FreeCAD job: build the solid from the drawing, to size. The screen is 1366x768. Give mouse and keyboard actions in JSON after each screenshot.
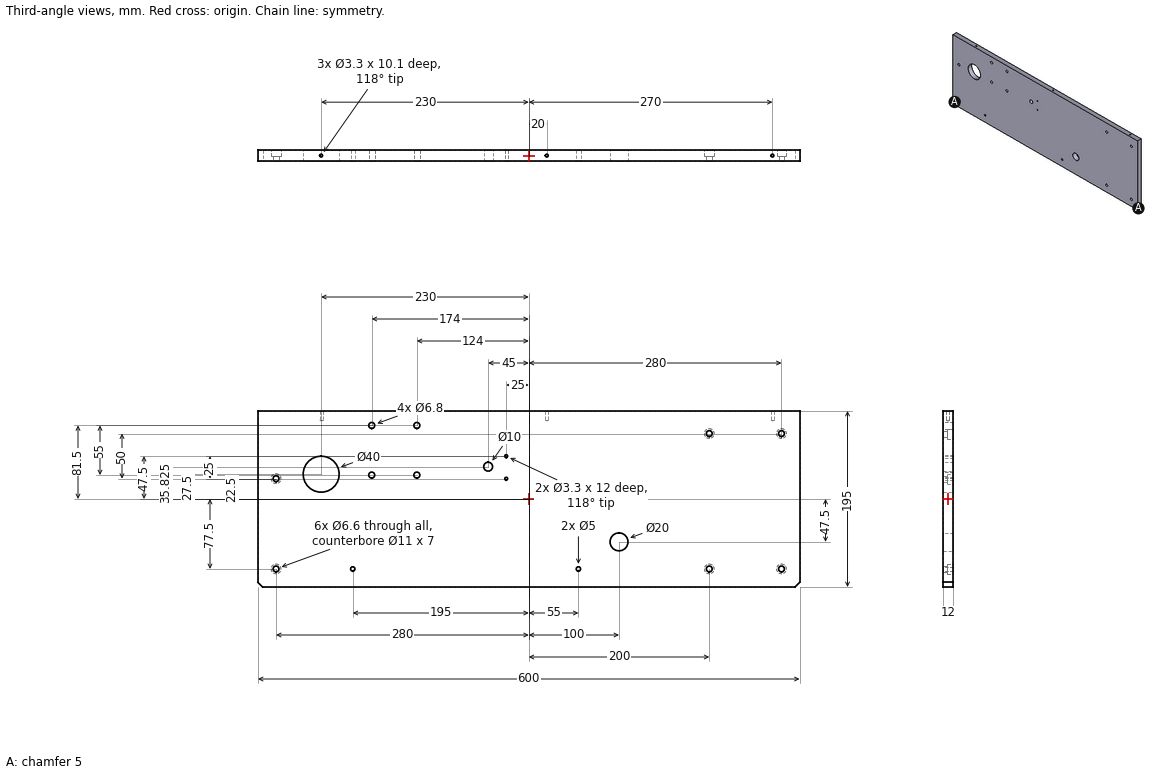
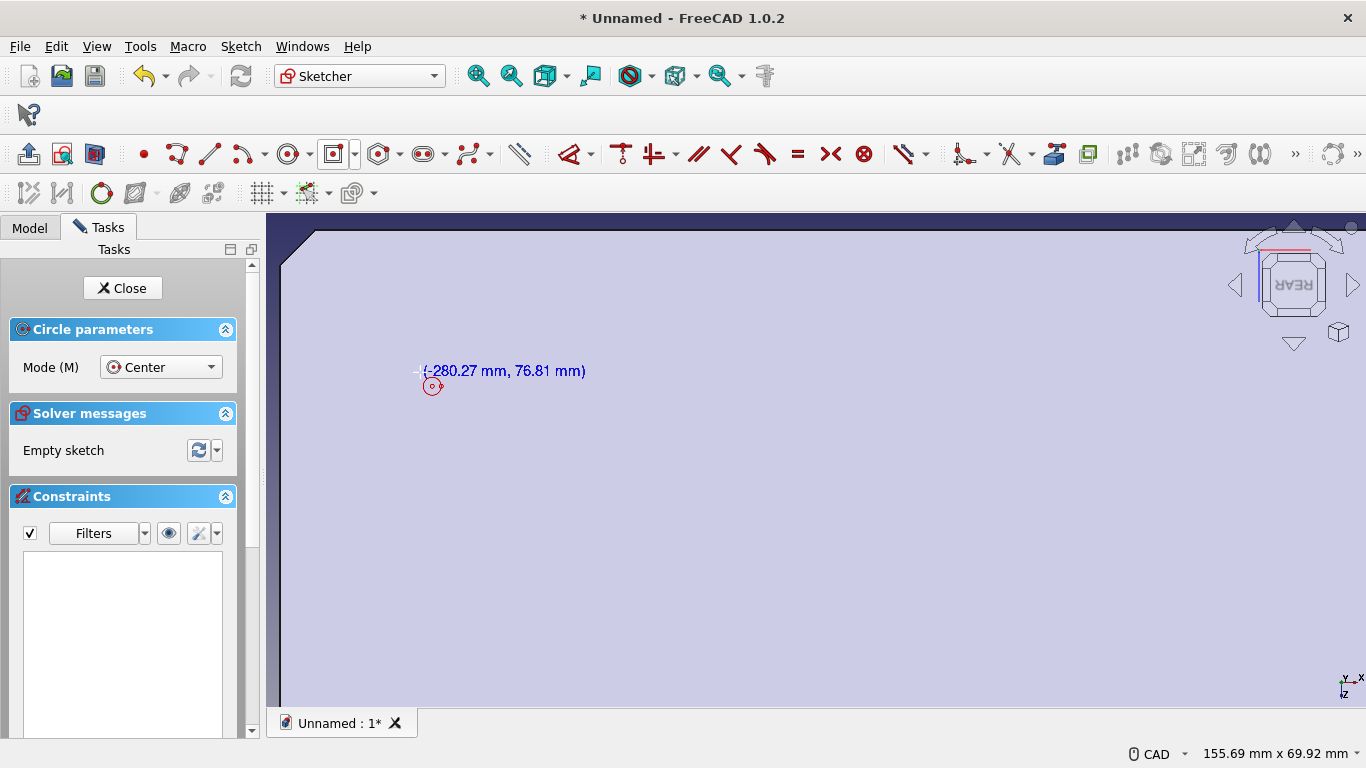
{"action": "scroll", "coordinate": [420, 373], "scroll_direction": "down", "scroll_amount": 9}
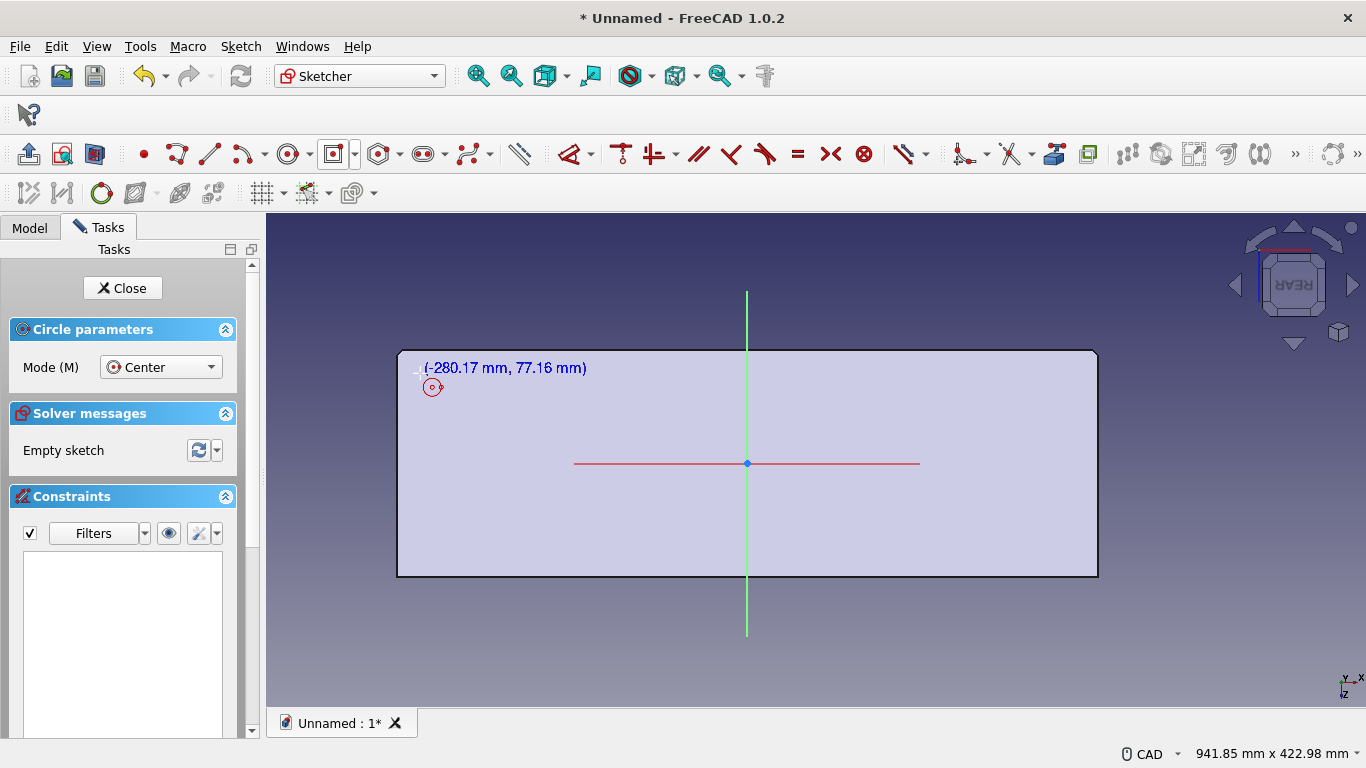
{"action": "left_click", "coordinate": [420, 373]}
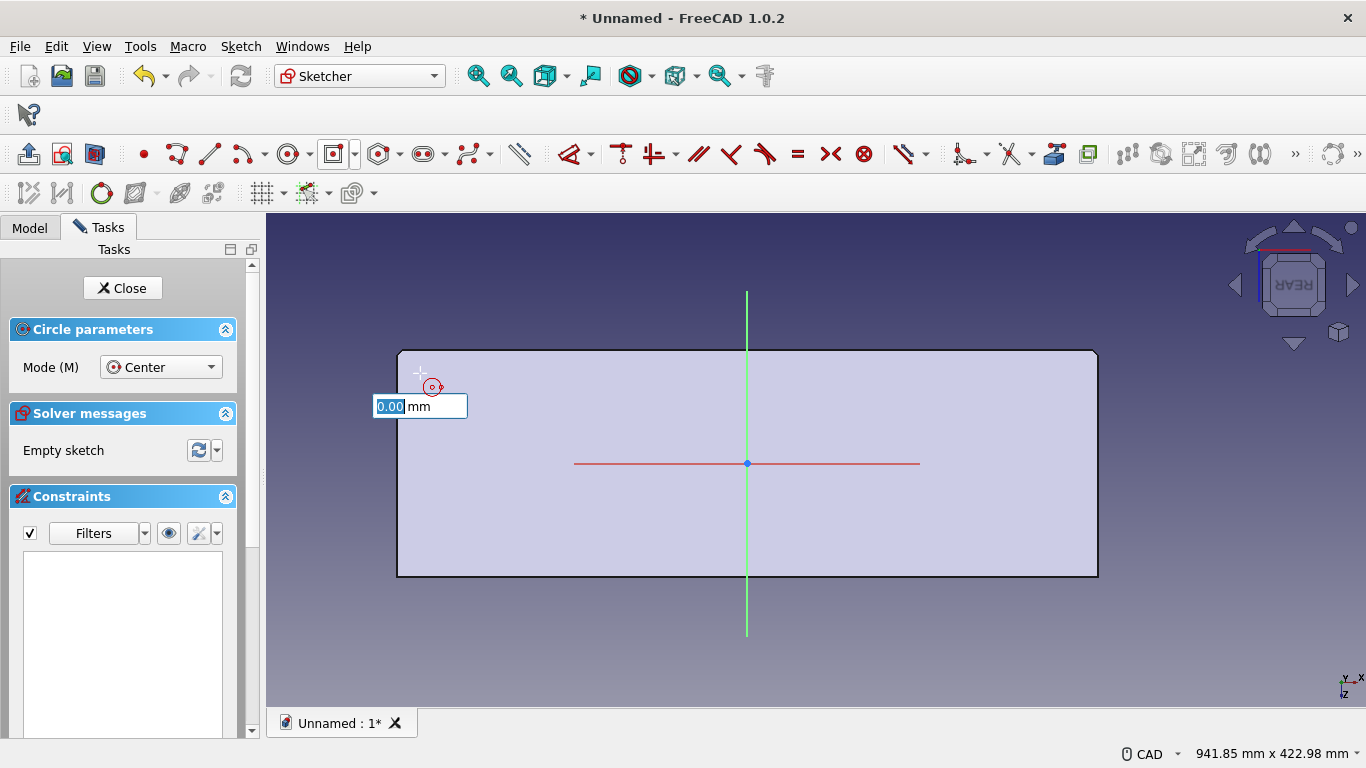
{"action": "scroll", "coordinate": [423, 370], "scroll_direction": "up", "scroll_amount": 8}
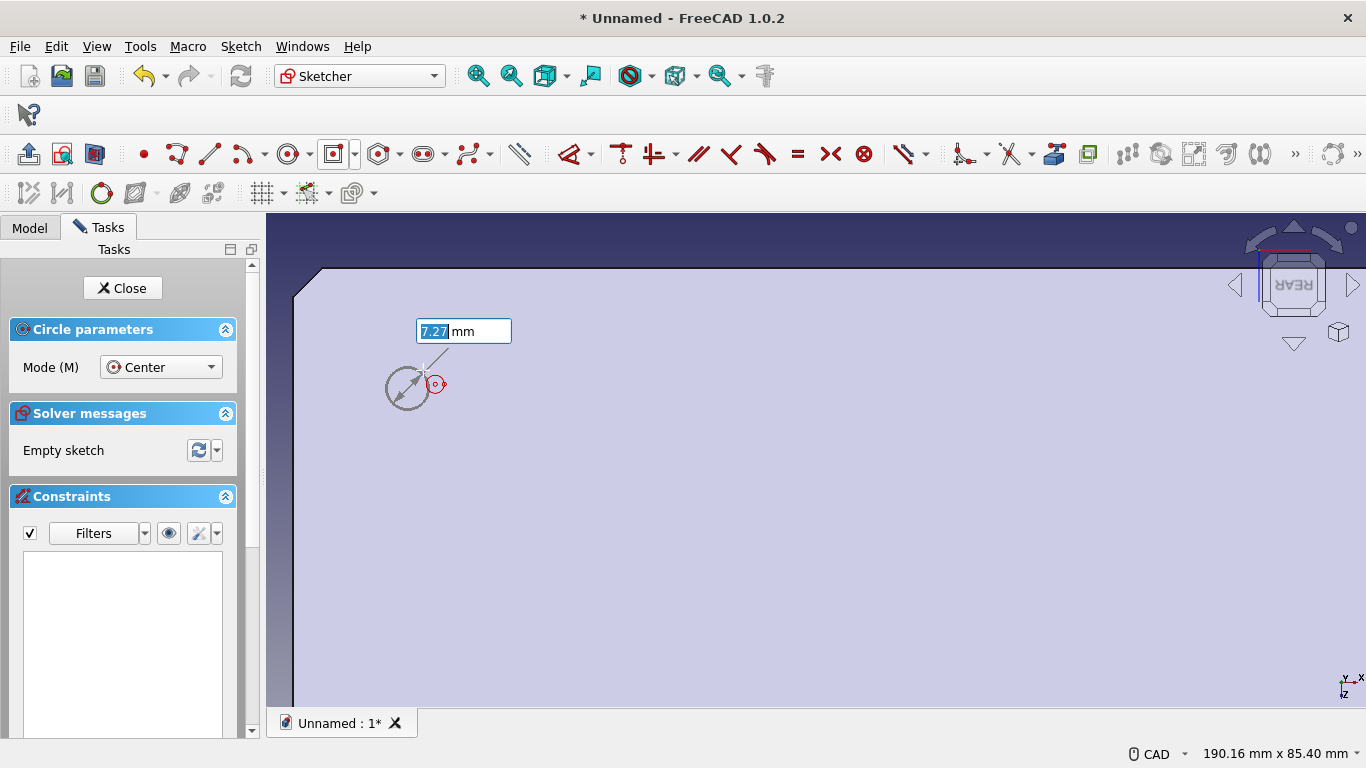
{"action": "left_click", "coordinate": [423, 370]}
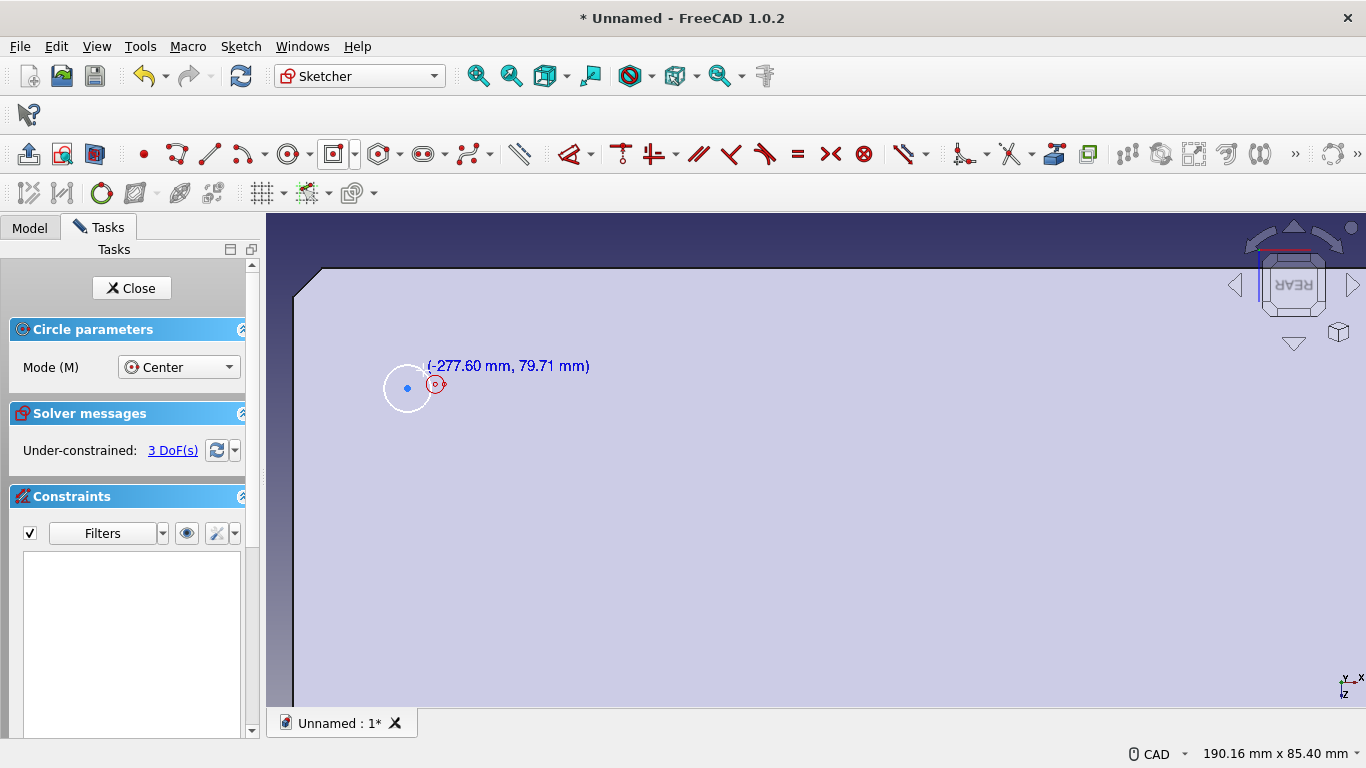
{"action": "scroll", "coordinate": [423, 370], "scroll_direction": "down", "scroll_amount": 8}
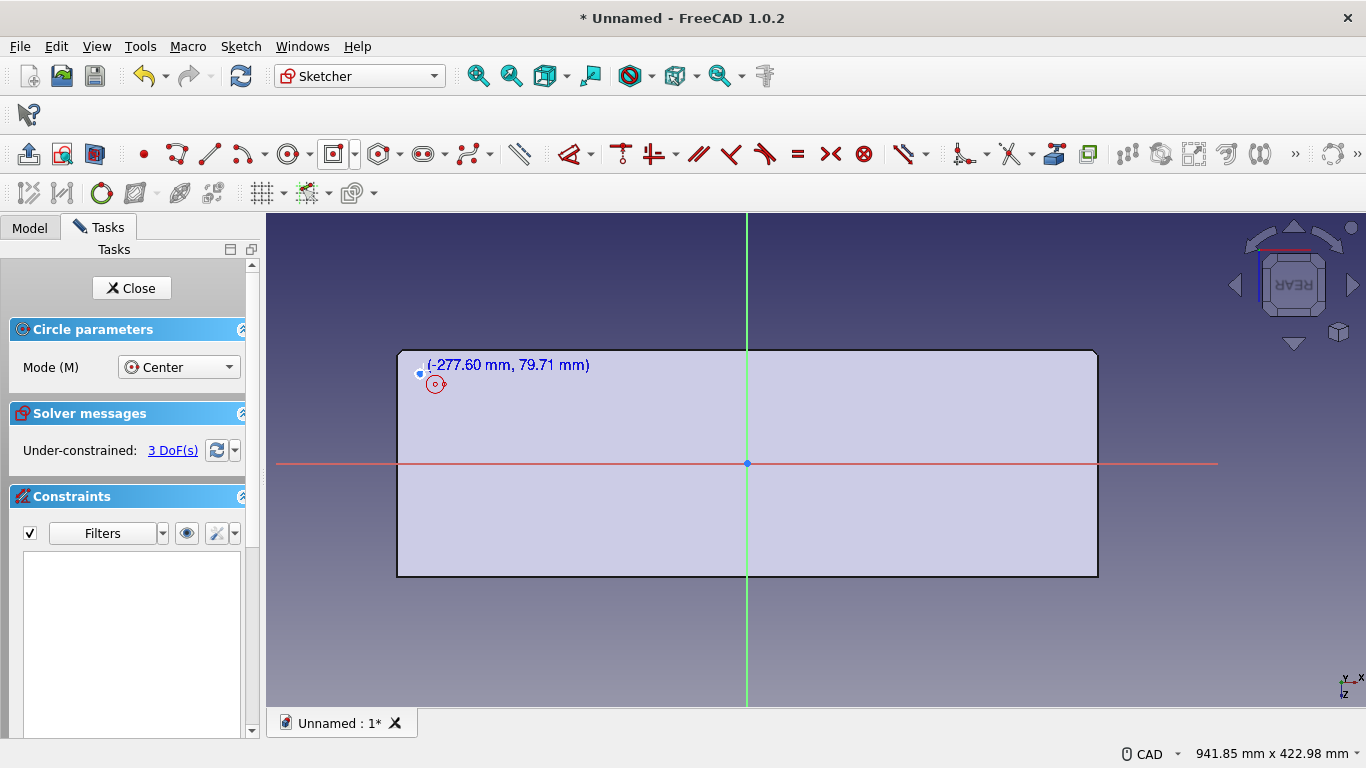
{"action": "scroll", "coordinate": [420, 490], "scroll_direction": "up", "scroll_amount": 9}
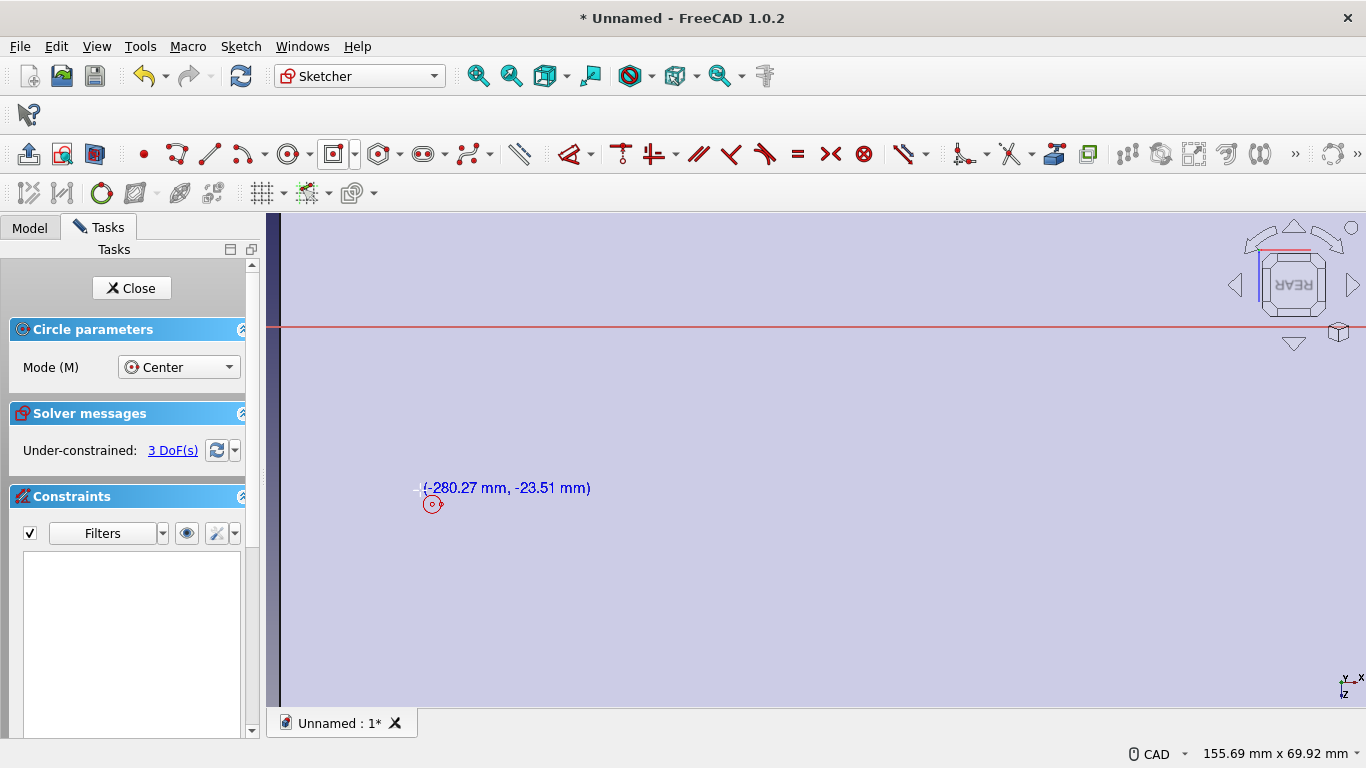
{"action": "scroll", "coordinate": [420, 490], "scroll_direction": "down", "scroll_amount": 9}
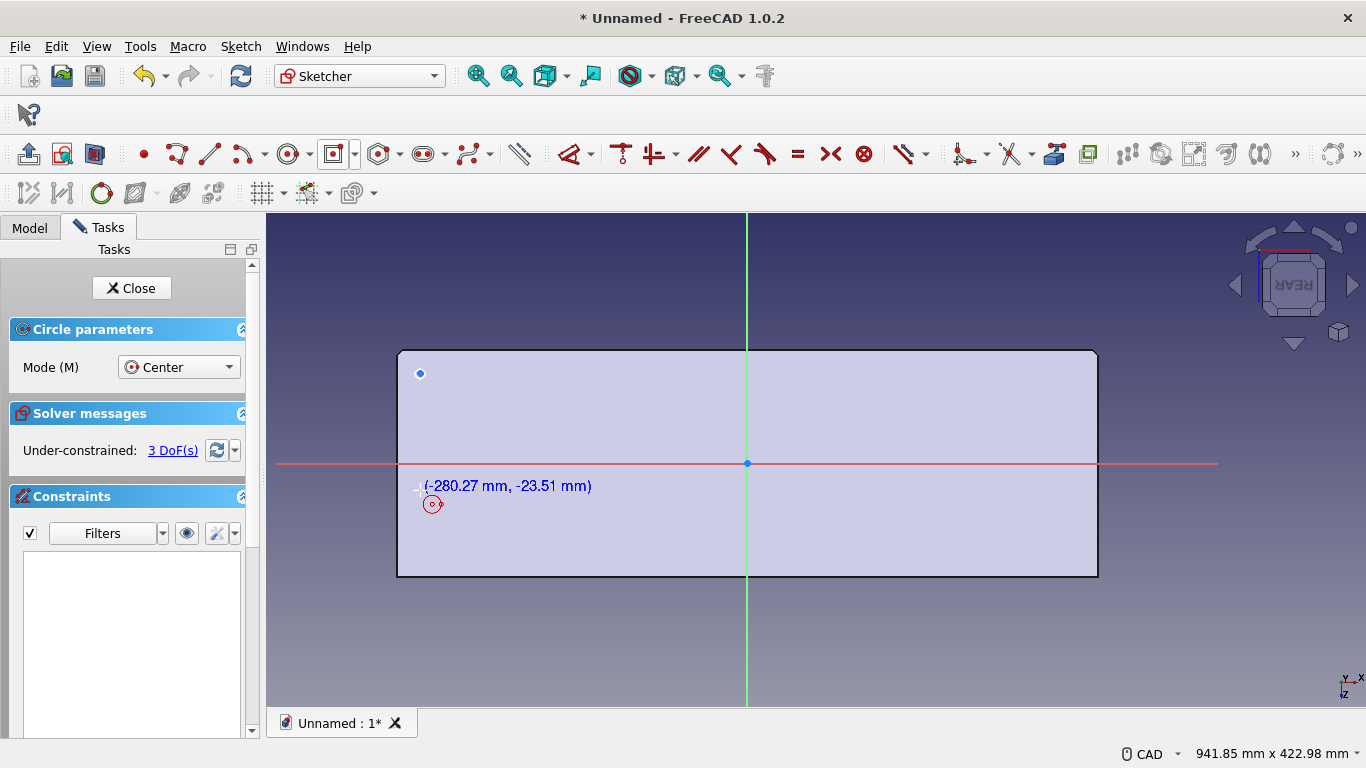
{"action": "left_click", "coordinate": [420, 490]}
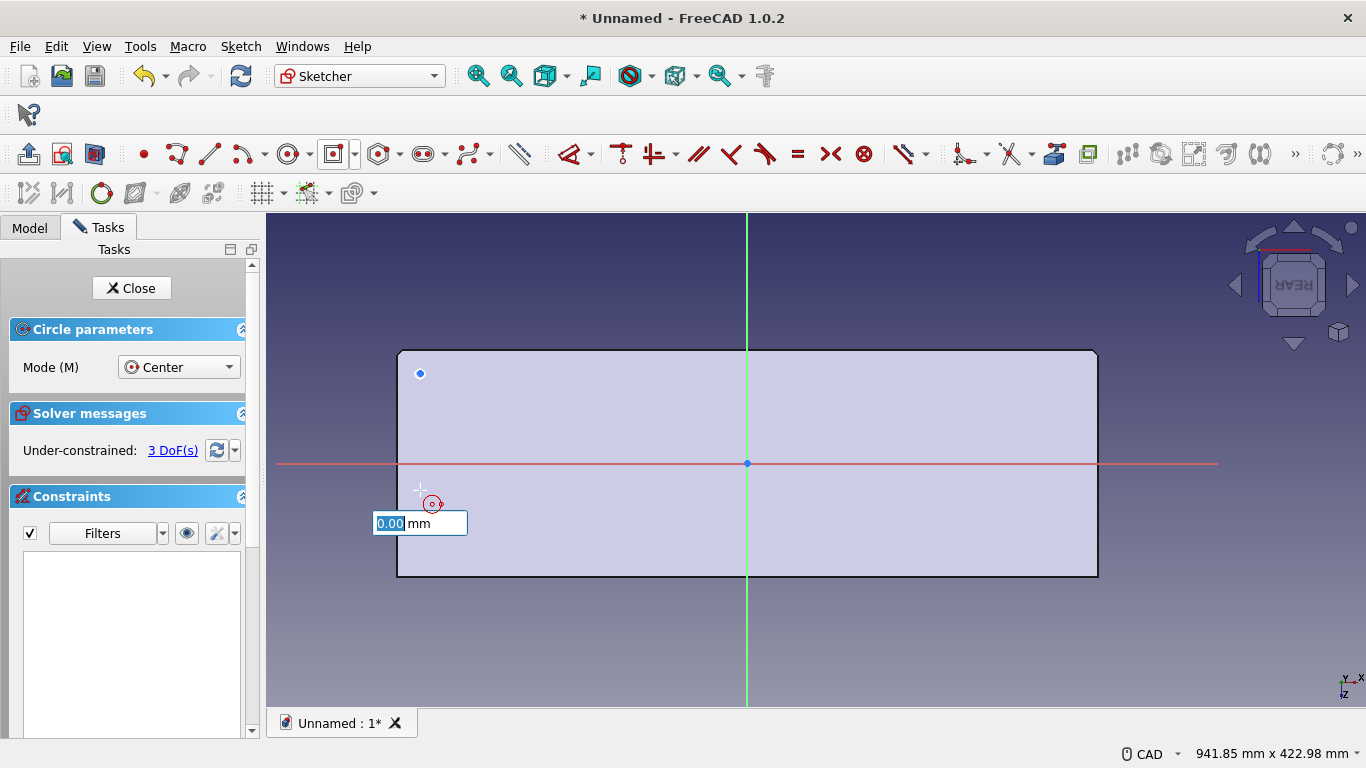
{"action": "scroll", "coordinate": [423, 487], "scroll_direction": "up", "scroll_amount": 8}